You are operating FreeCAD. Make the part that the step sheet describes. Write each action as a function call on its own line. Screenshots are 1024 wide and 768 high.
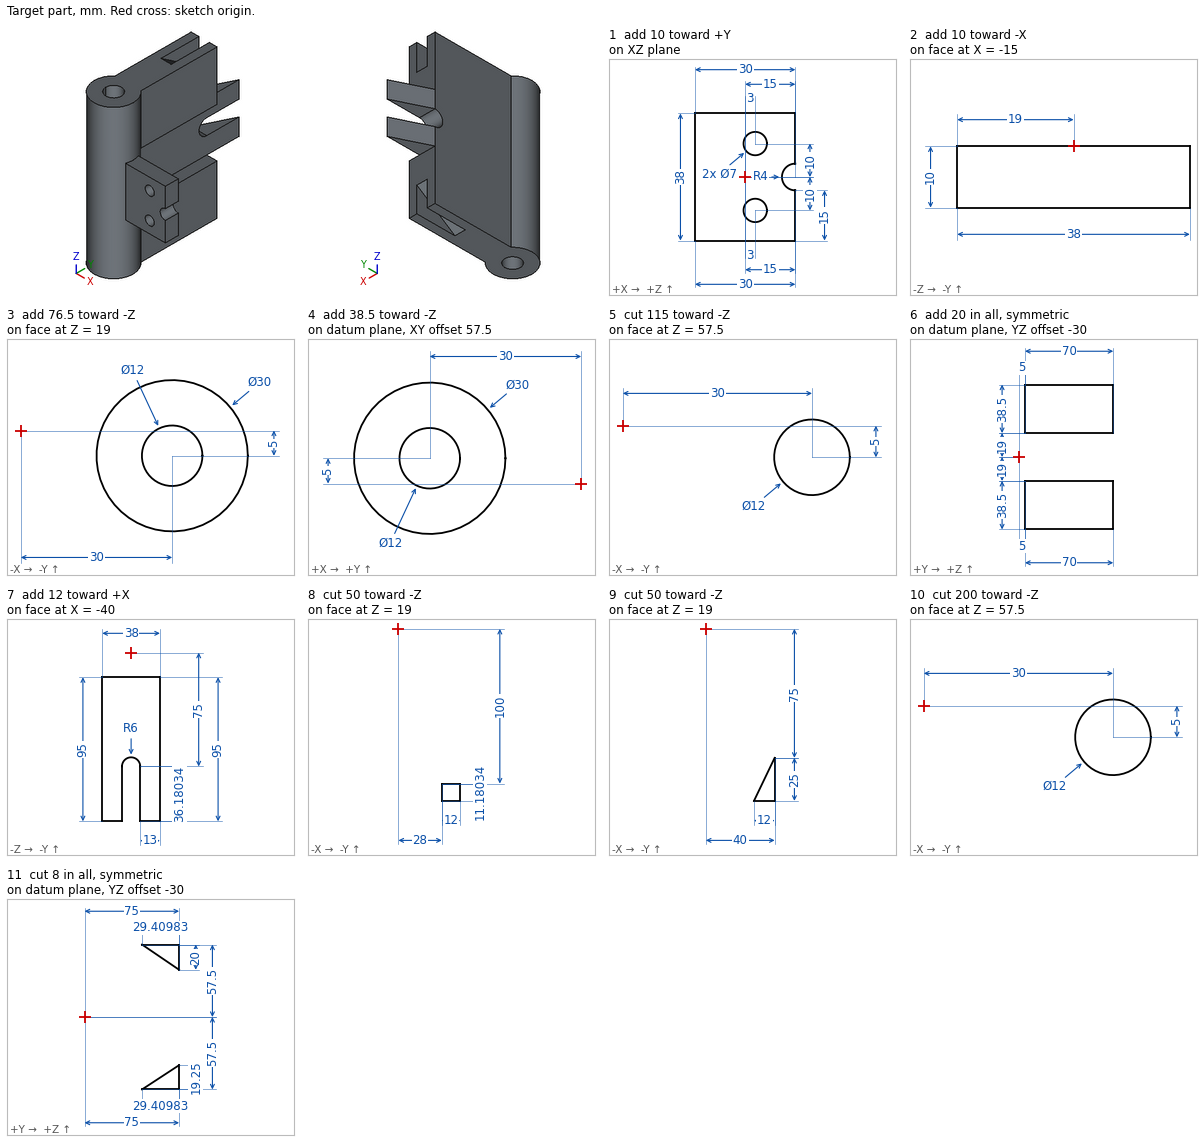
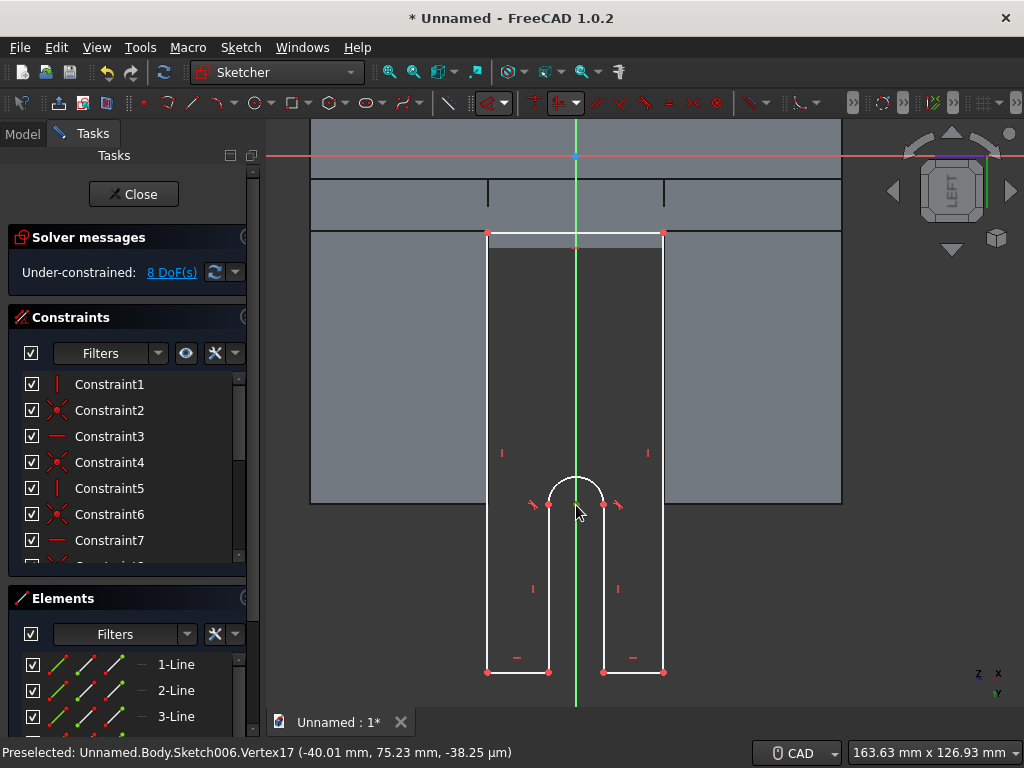
click(576, 413)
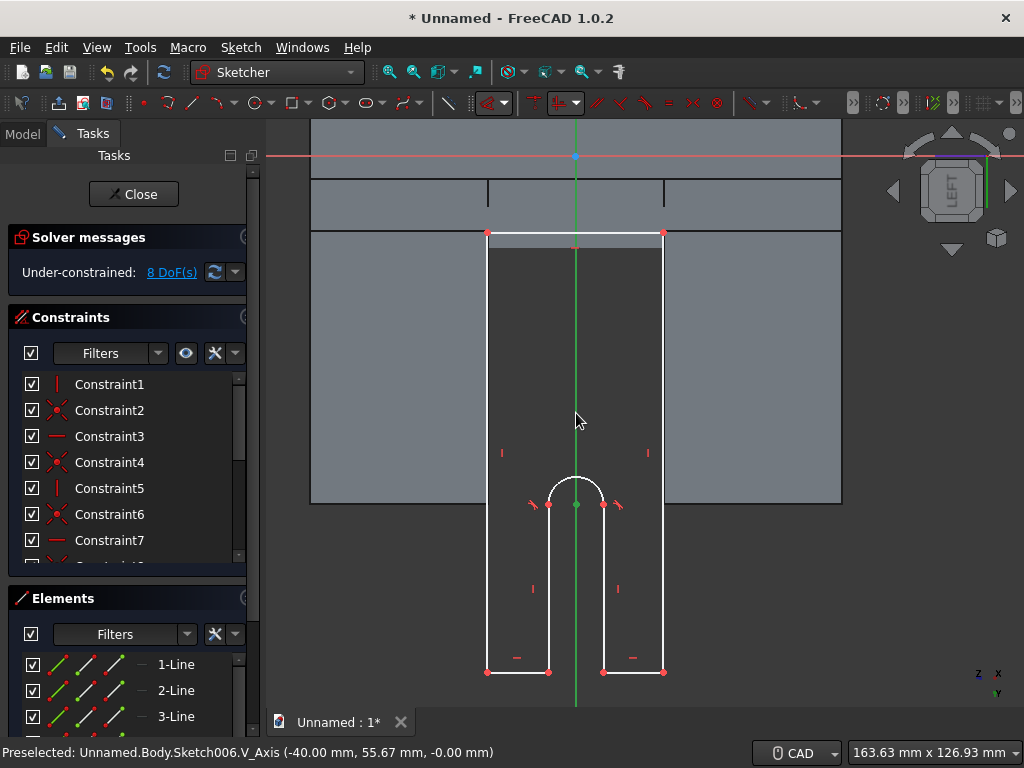
click(534, 104)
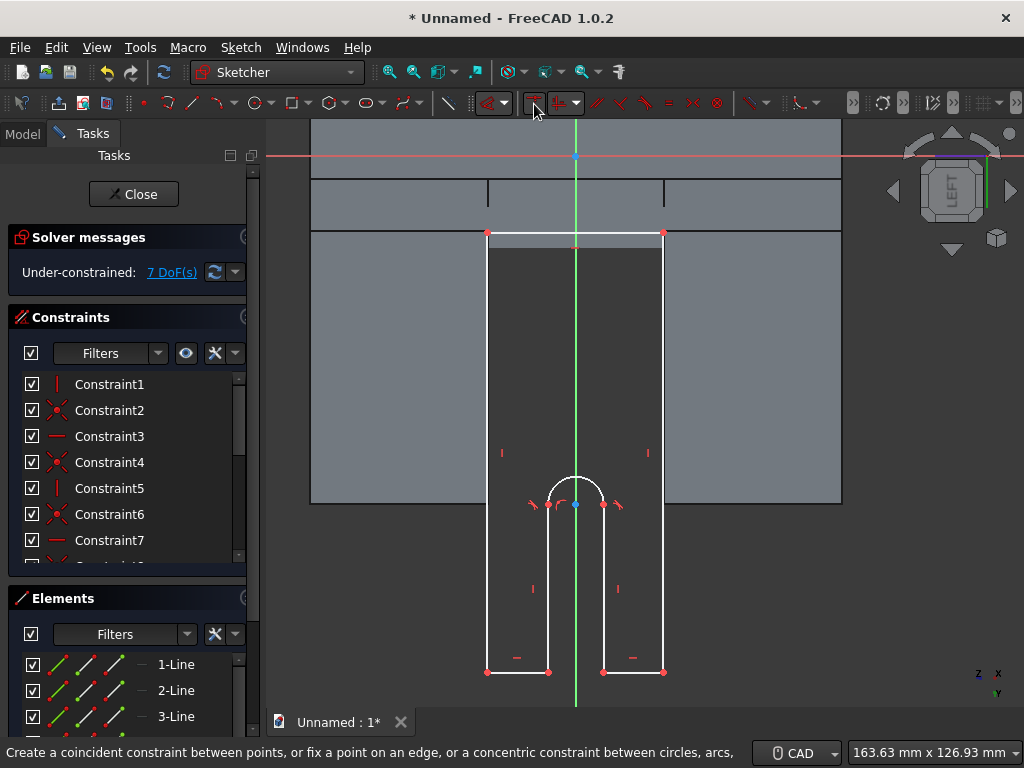
scroll(592, 482, up, 2)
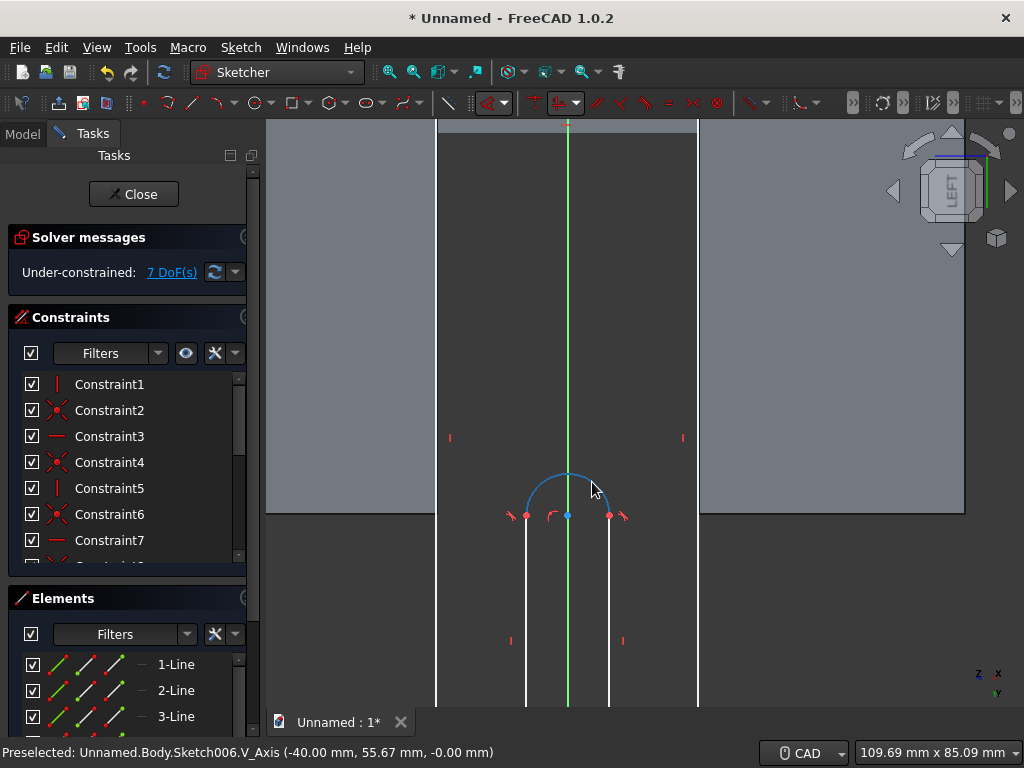
click(592, 482)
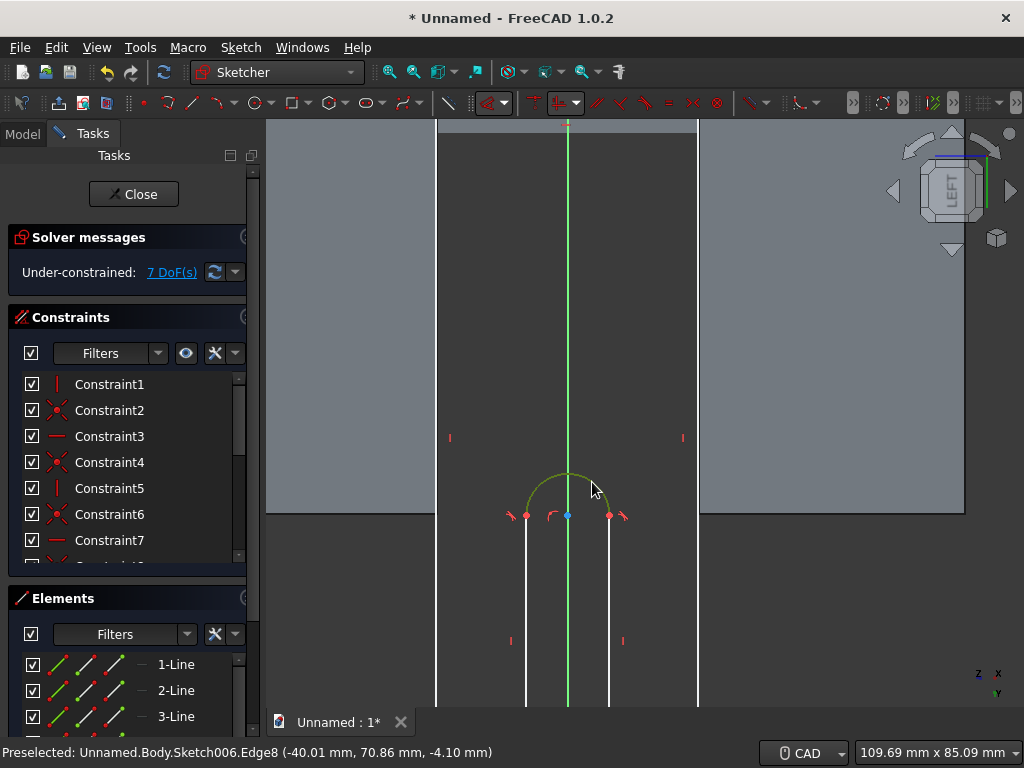
key(k)
key(r)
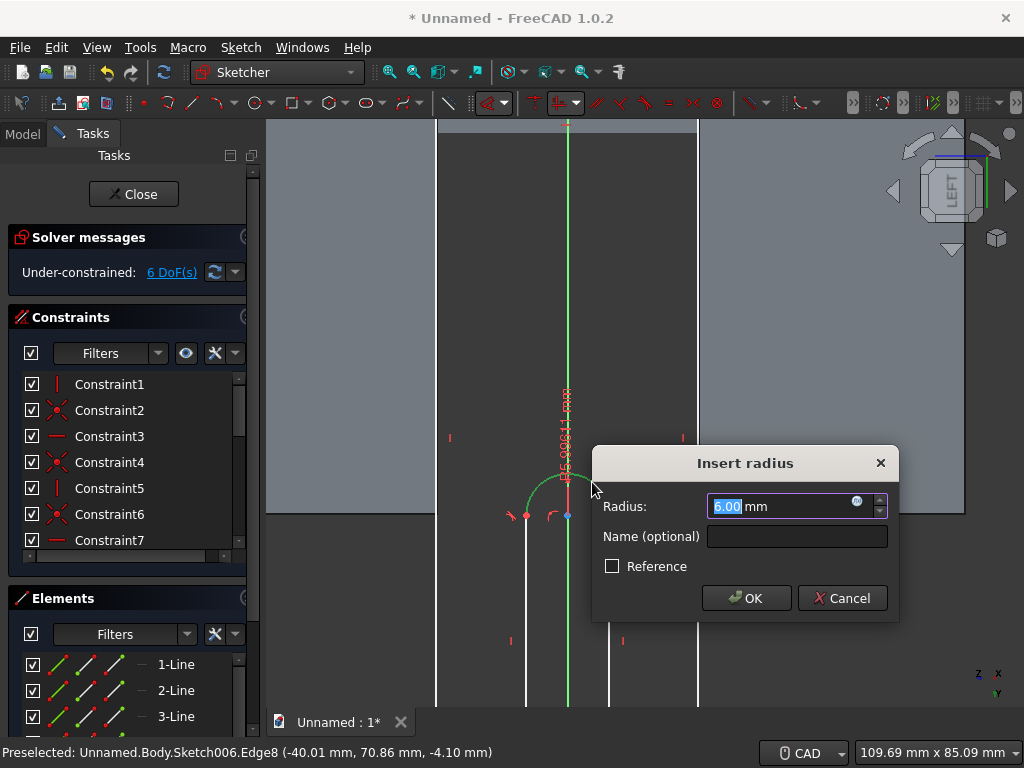
text(6)
key(Return)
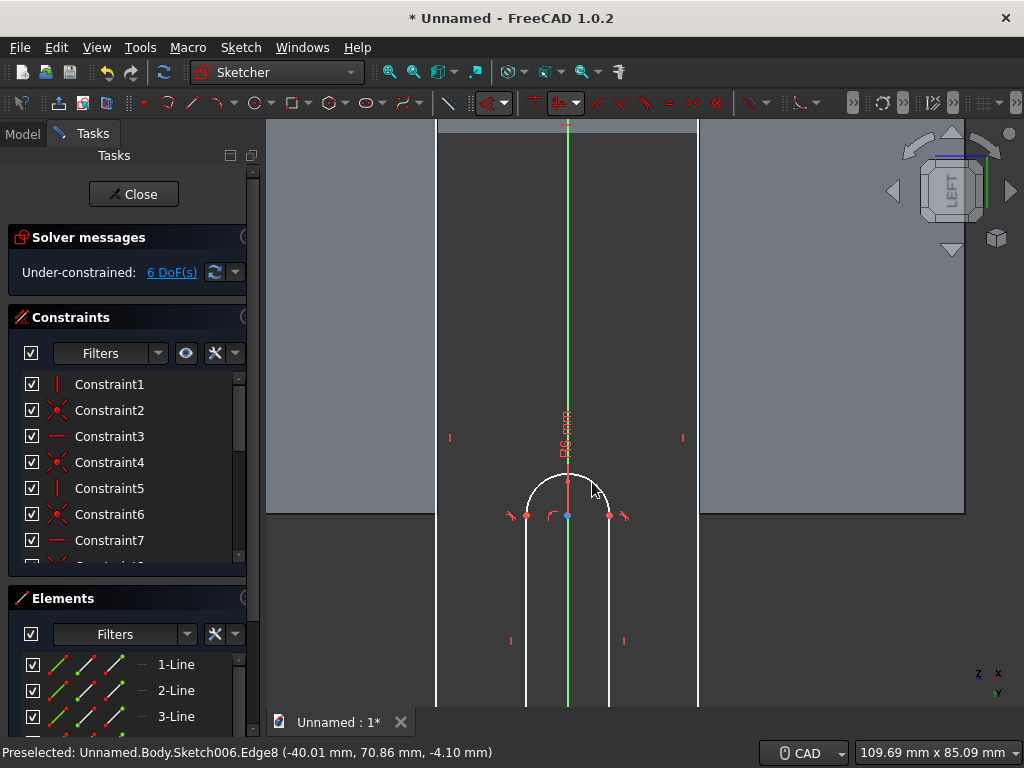
scroll(584, 440, down, 4)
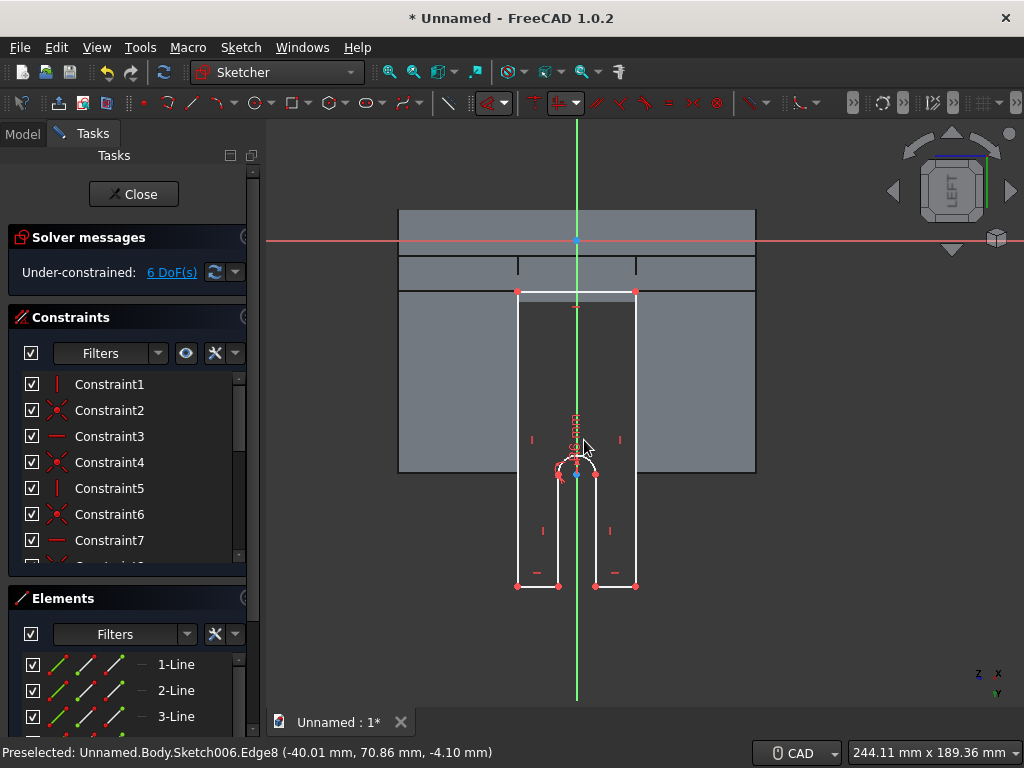
click(608, 587)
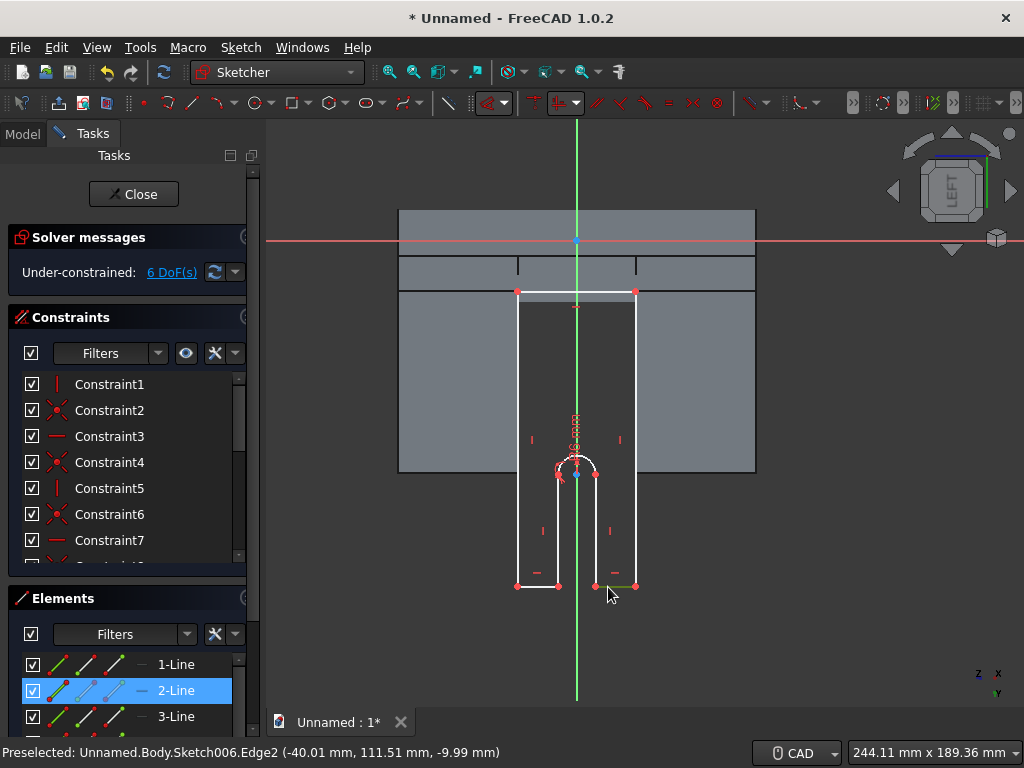
click(506, 104)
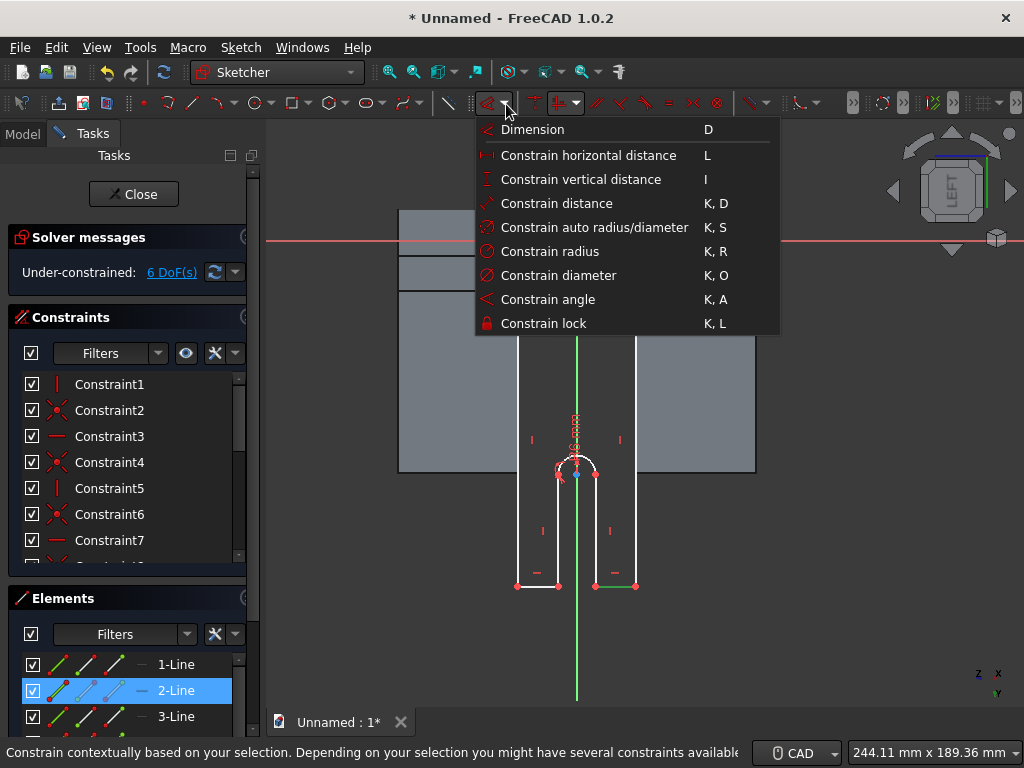
click(628, 155)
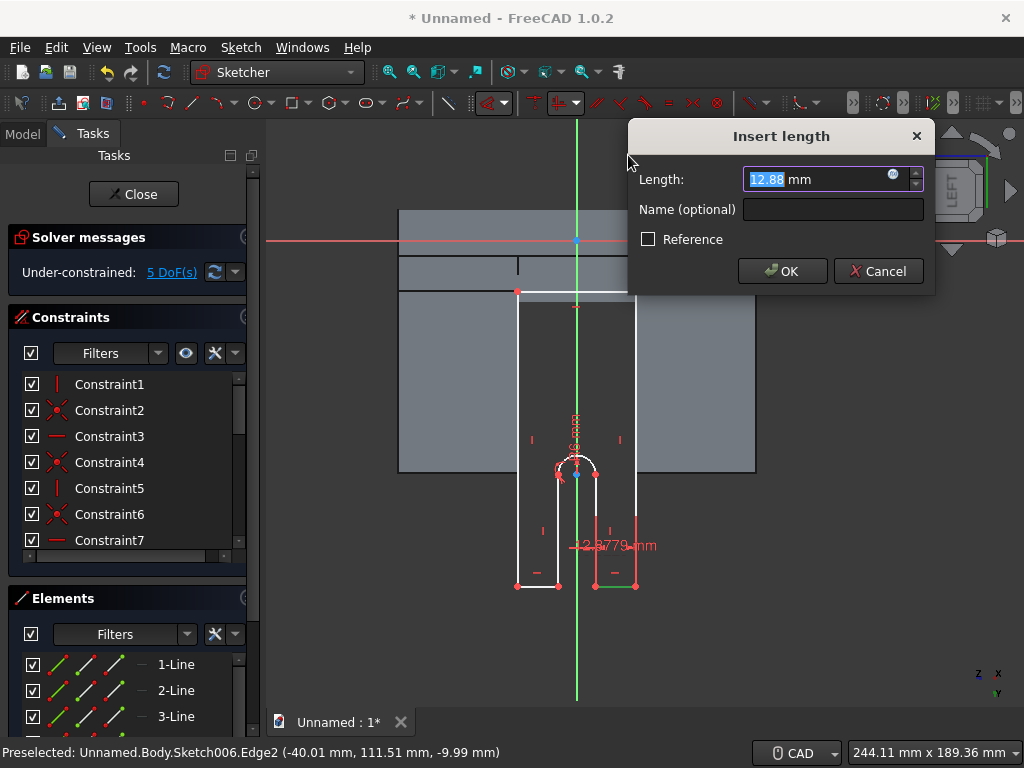
text(13)
key(Return)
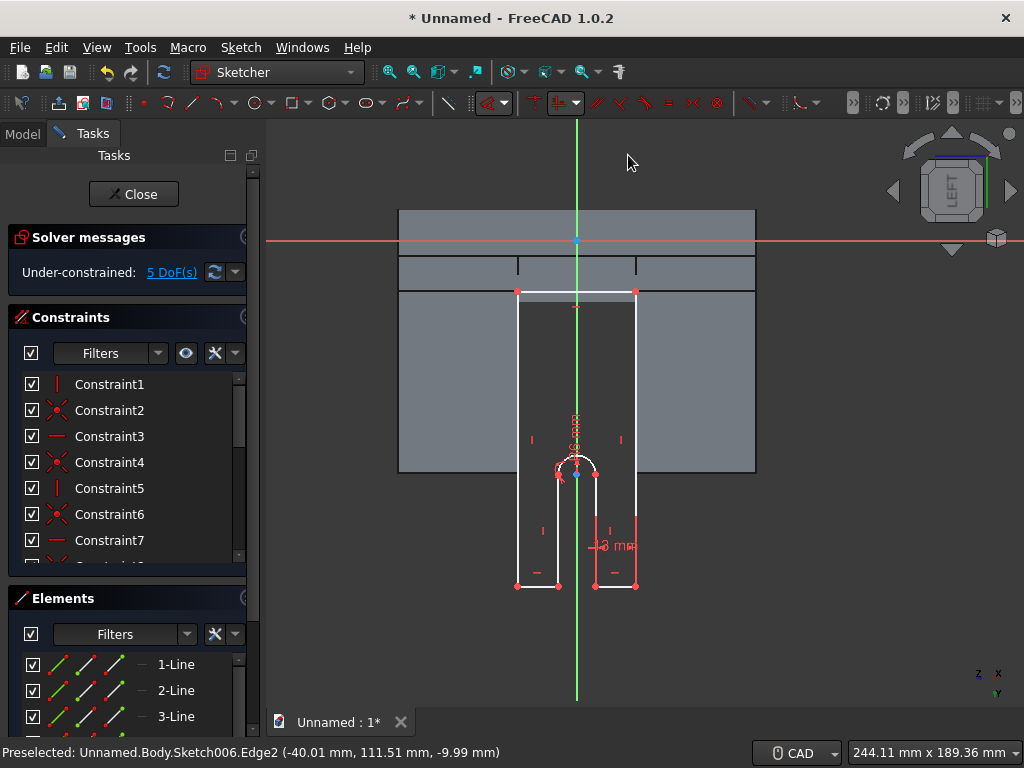
click(636, 498)